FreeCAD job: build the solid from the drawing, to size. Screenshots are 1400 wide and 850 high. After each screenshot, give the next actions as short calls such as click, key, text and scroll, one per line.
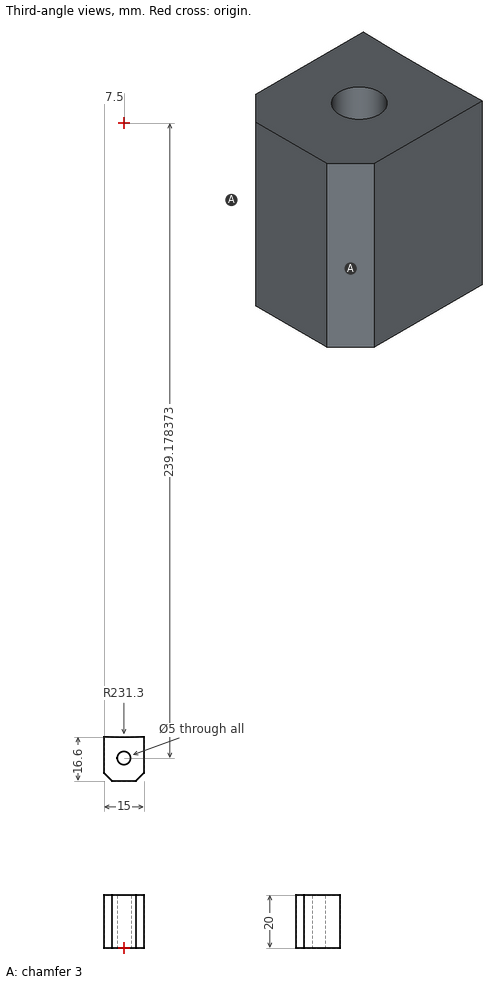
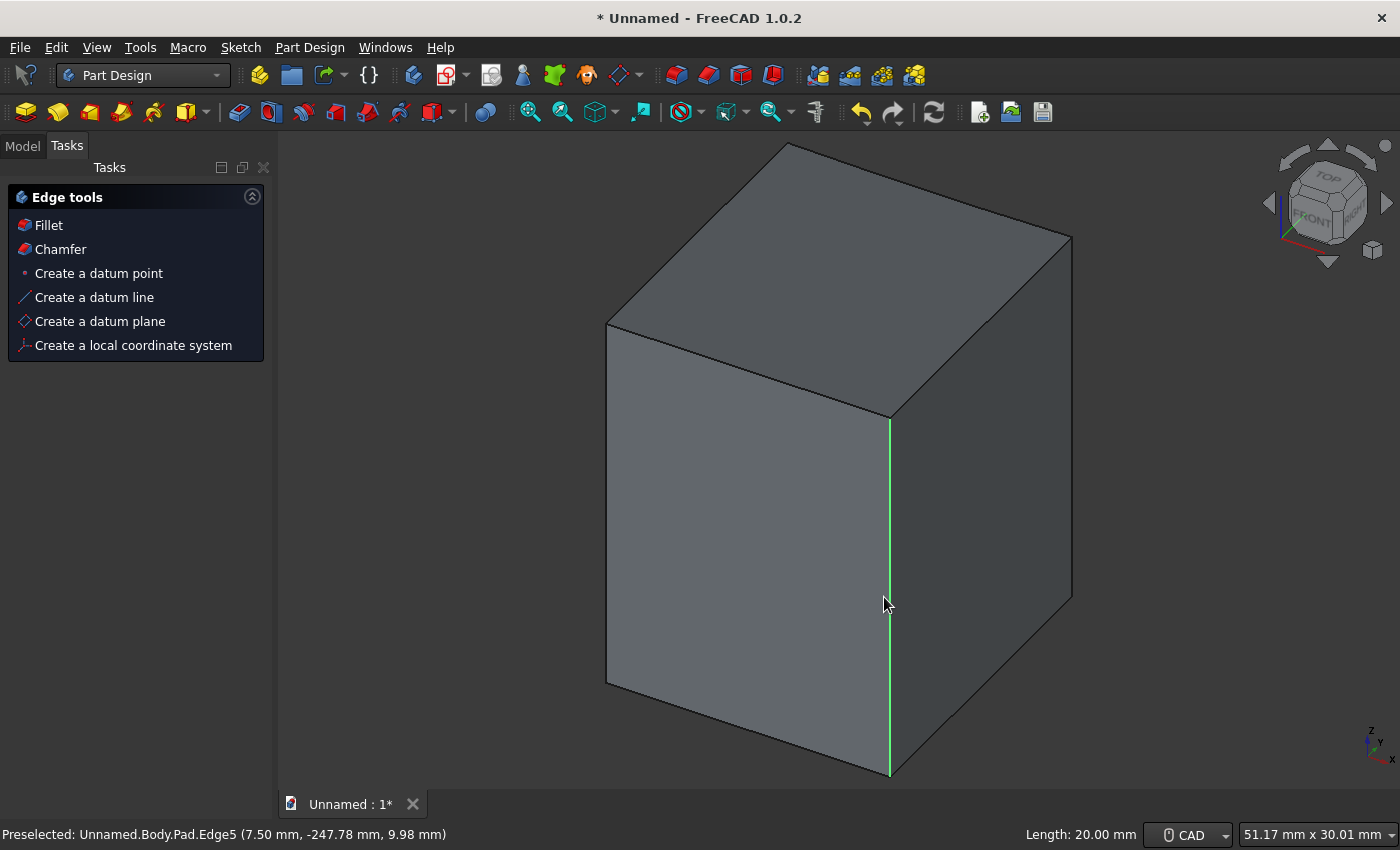
key(0)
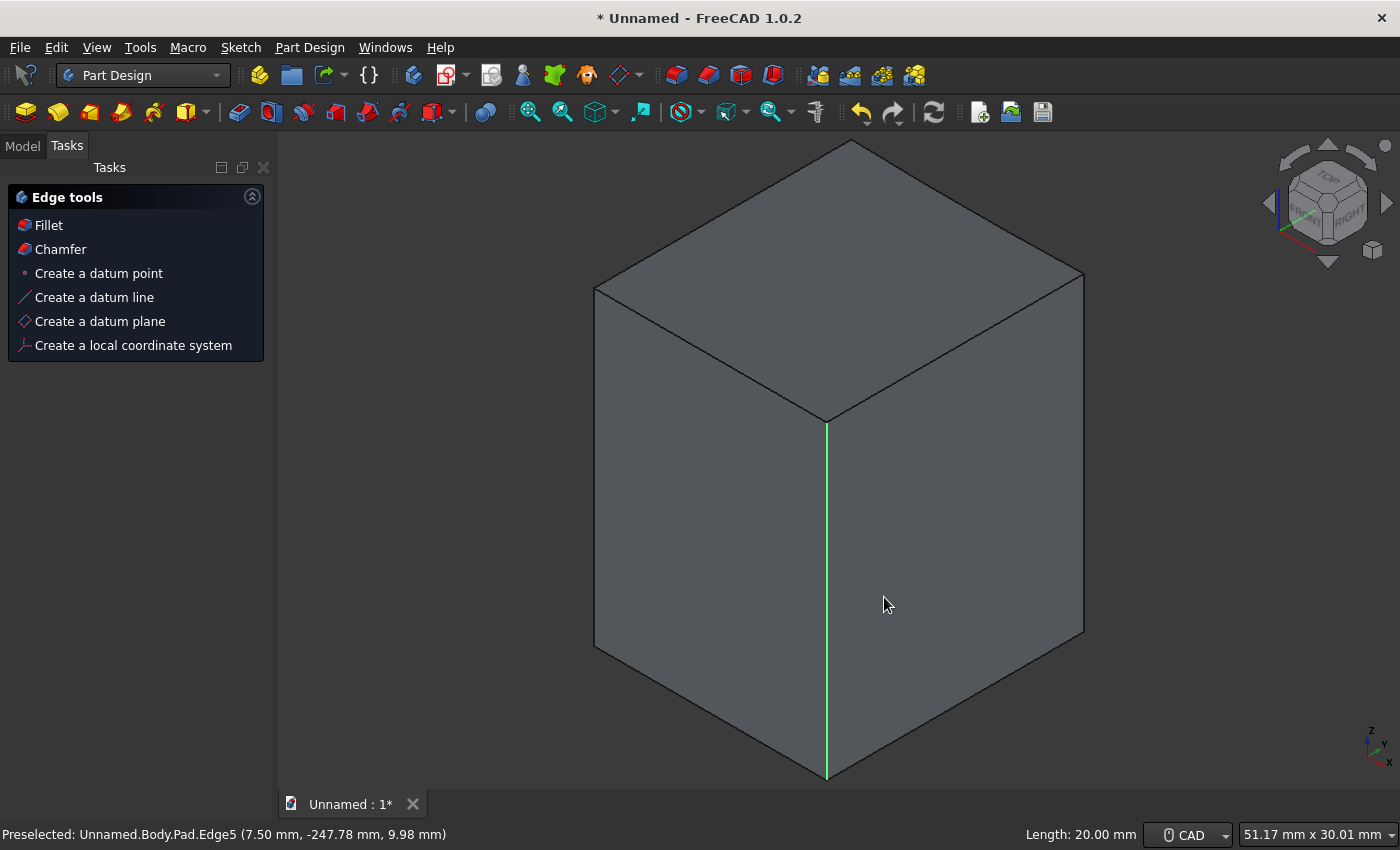
key(2)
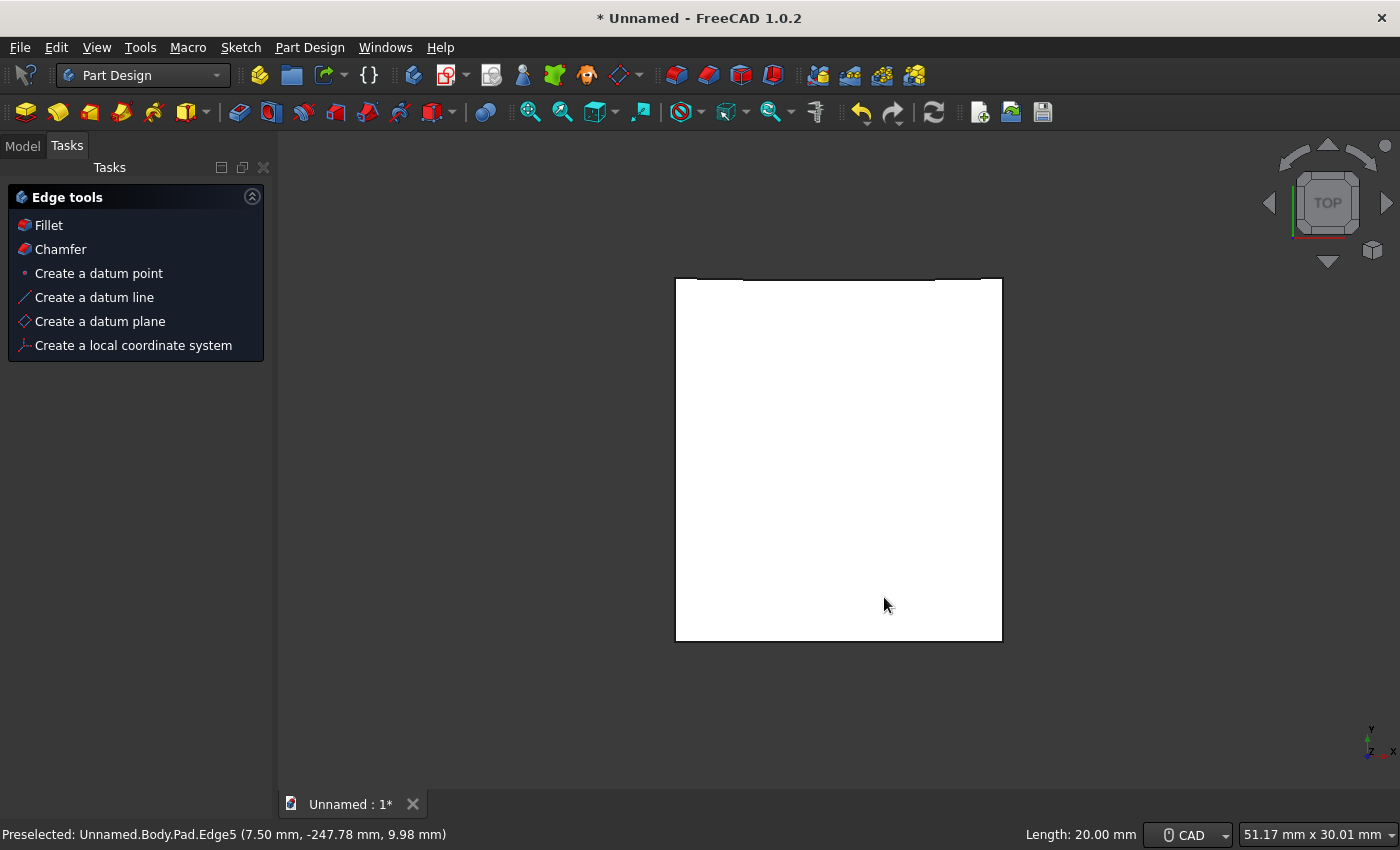
key(1)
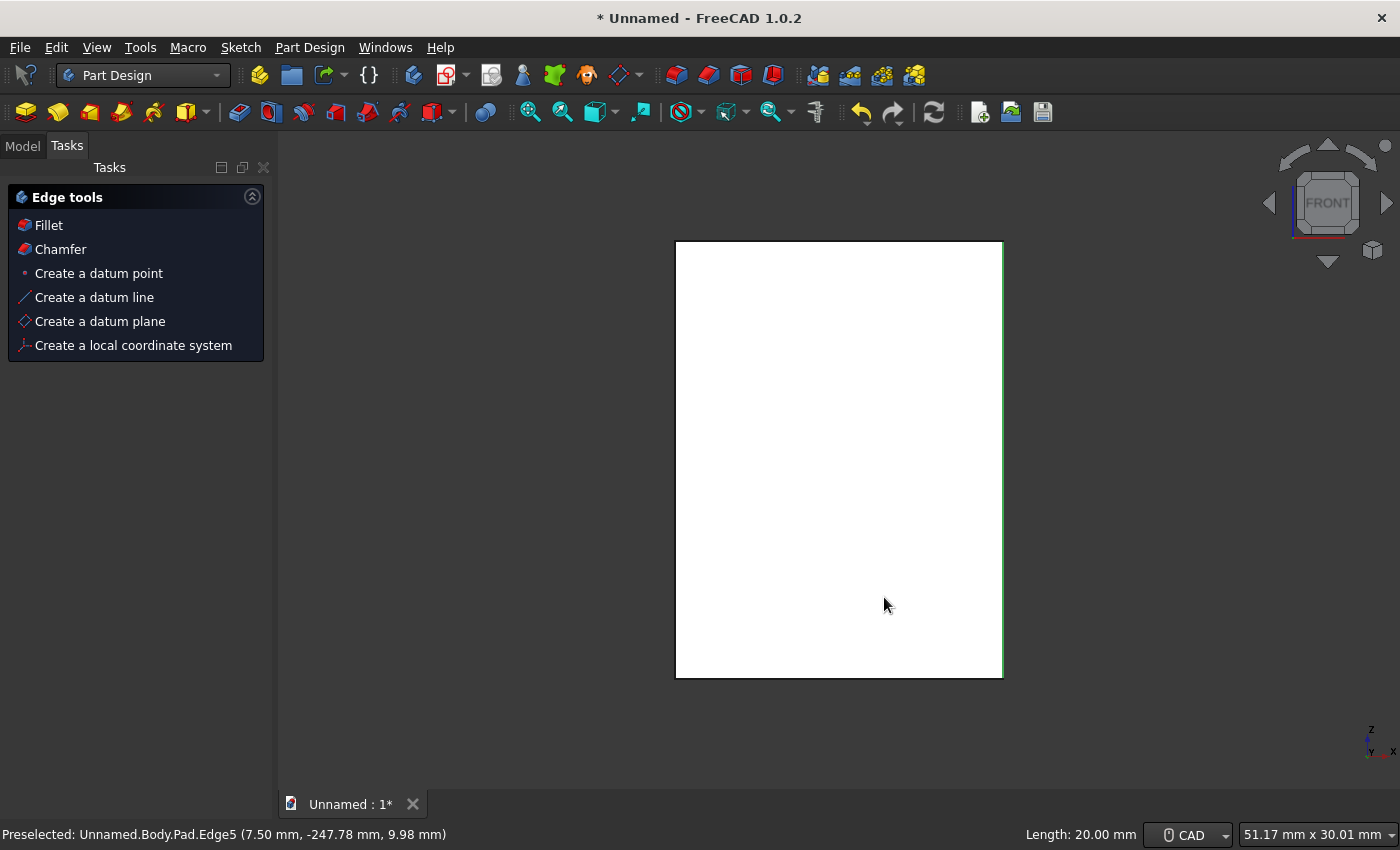
click(675, 459, ctrl)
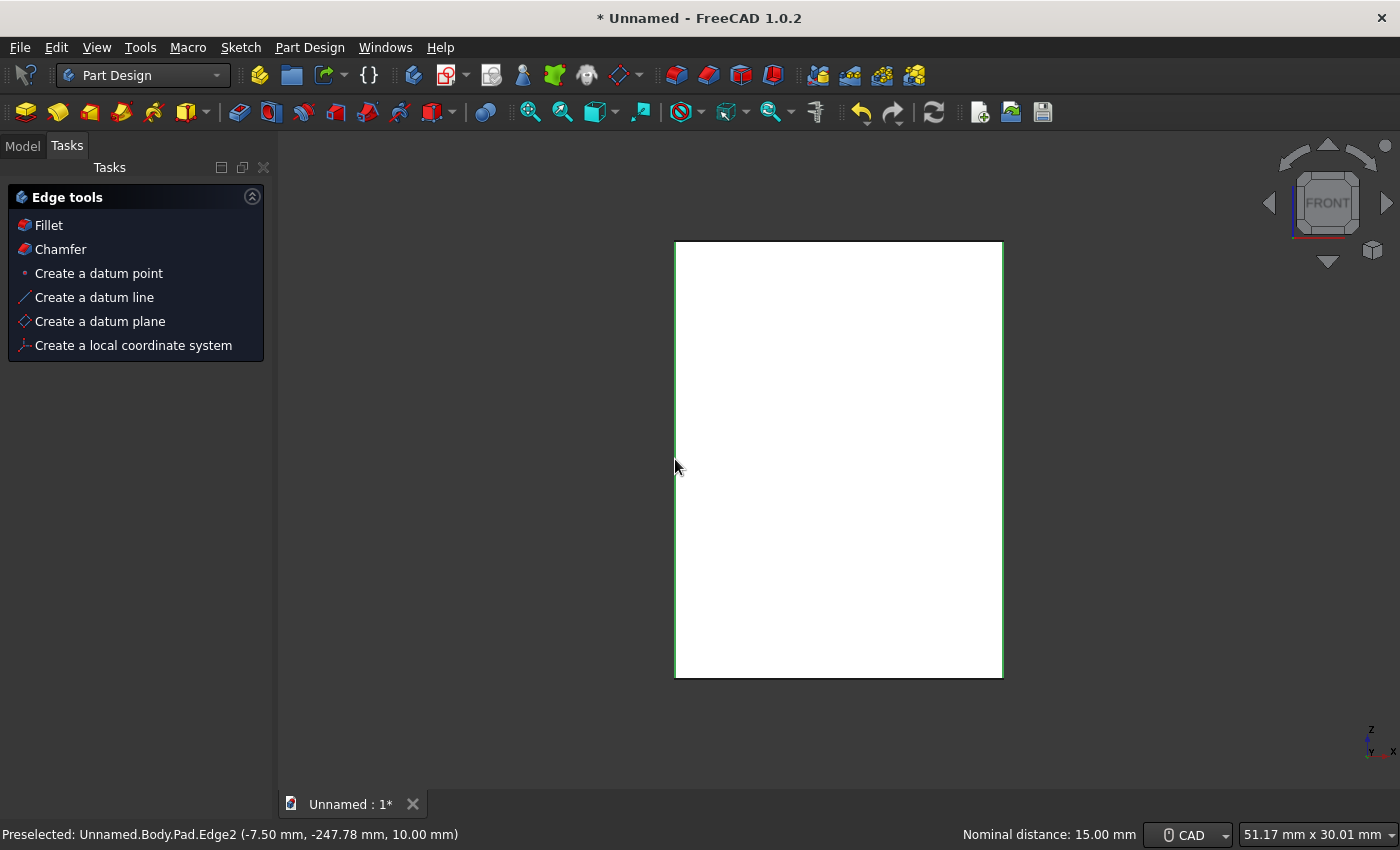
click(710, 76)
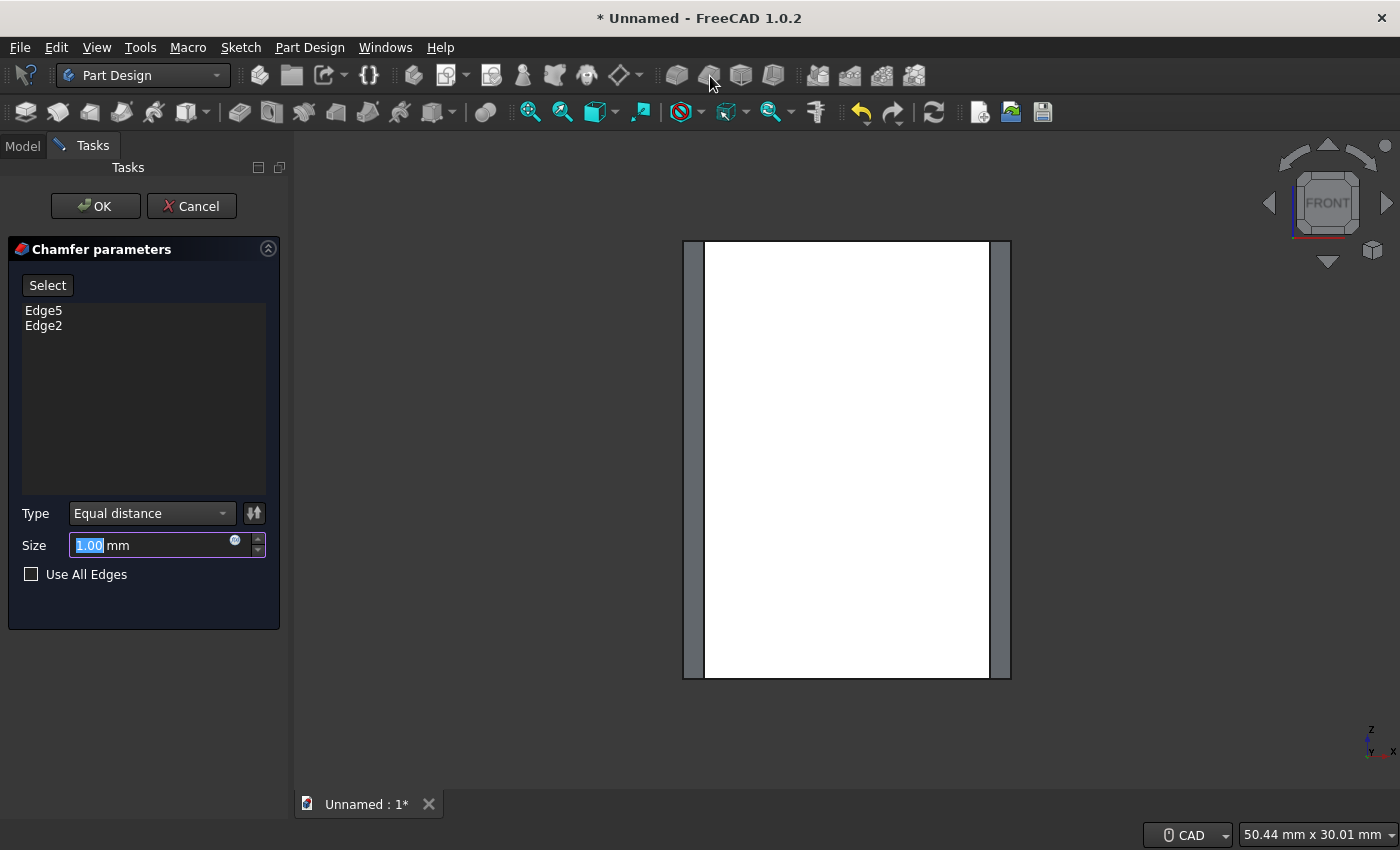
text(3)
key(Tab)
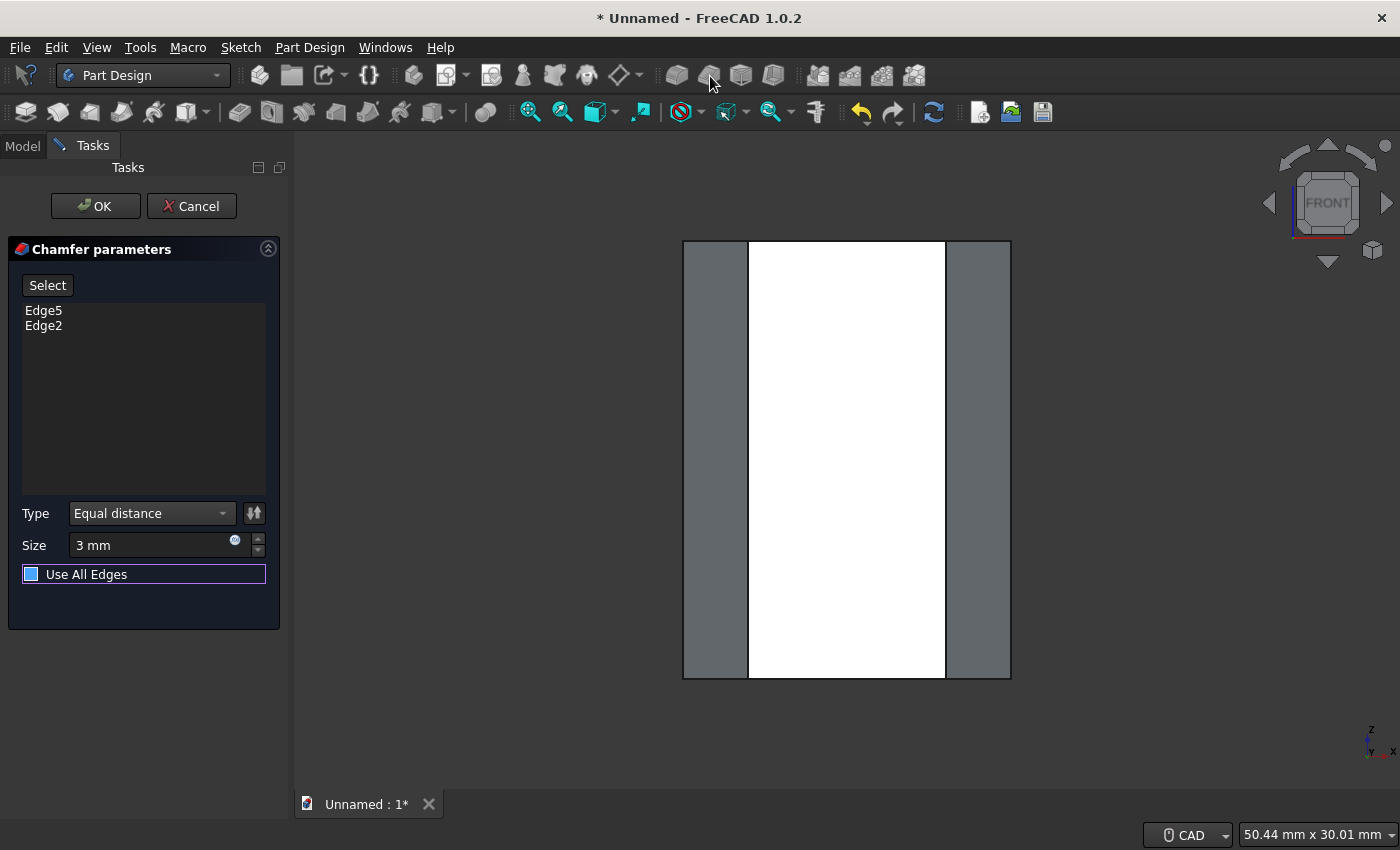
click(96, 206)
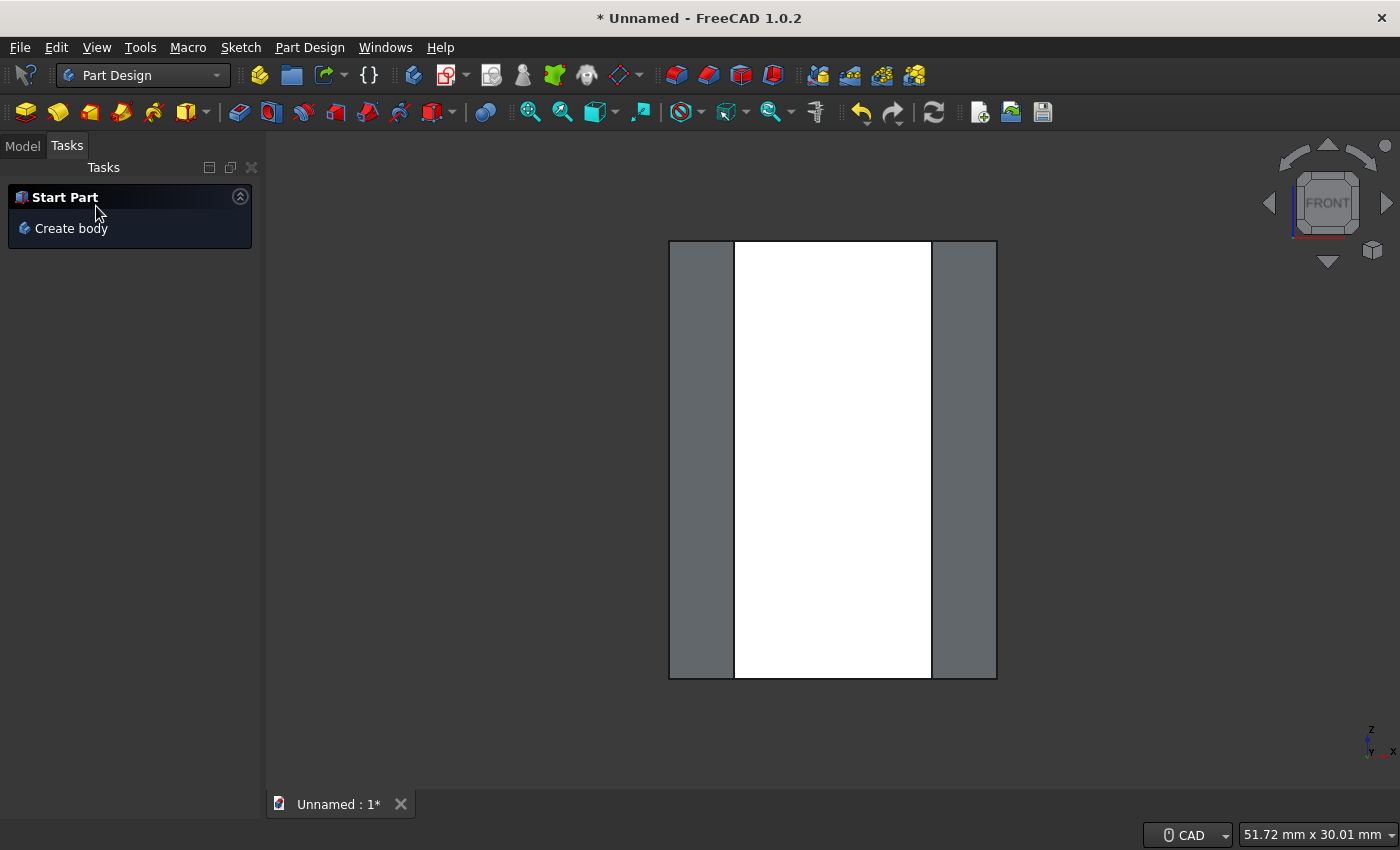
key(0)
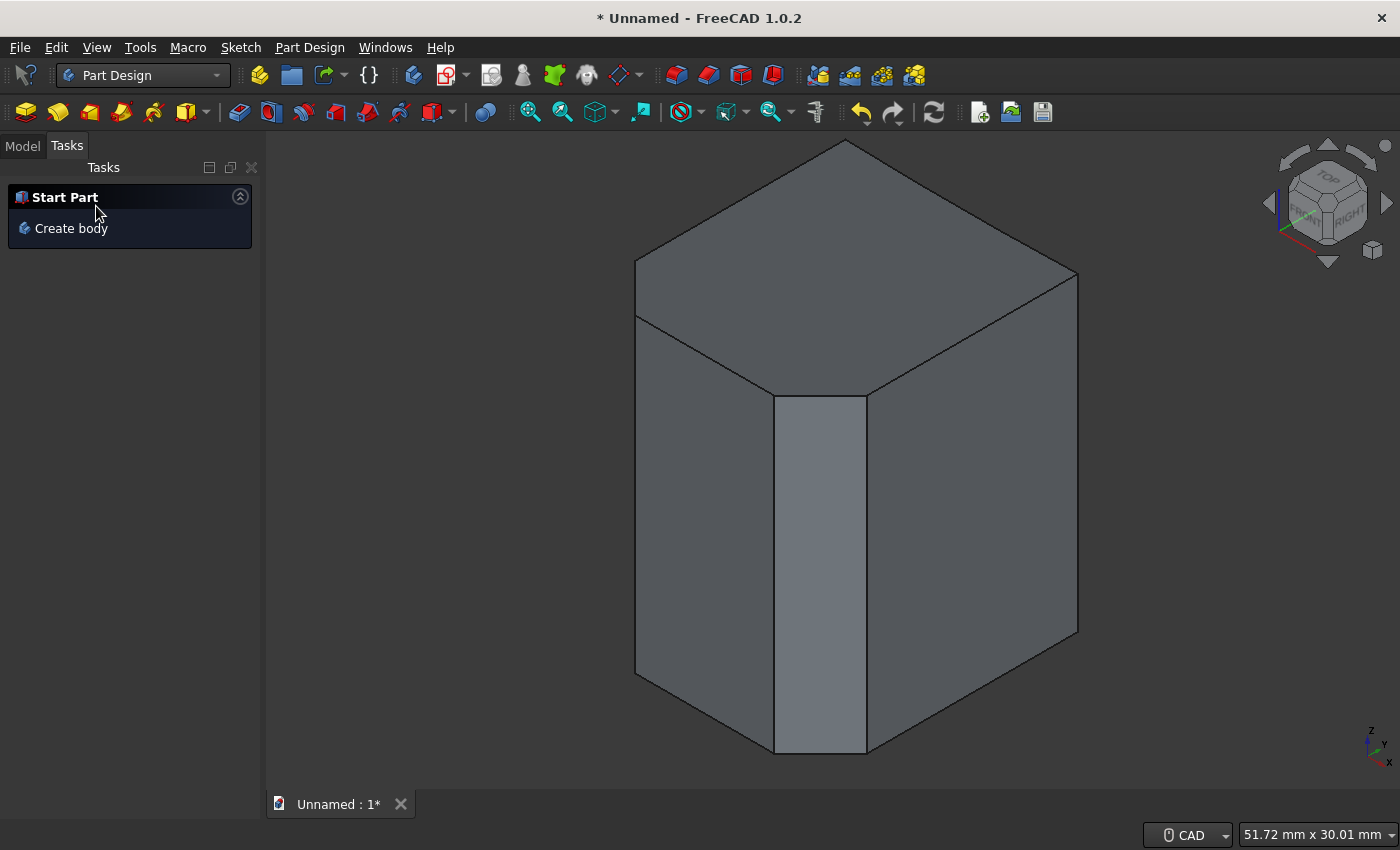
click(833, 280)